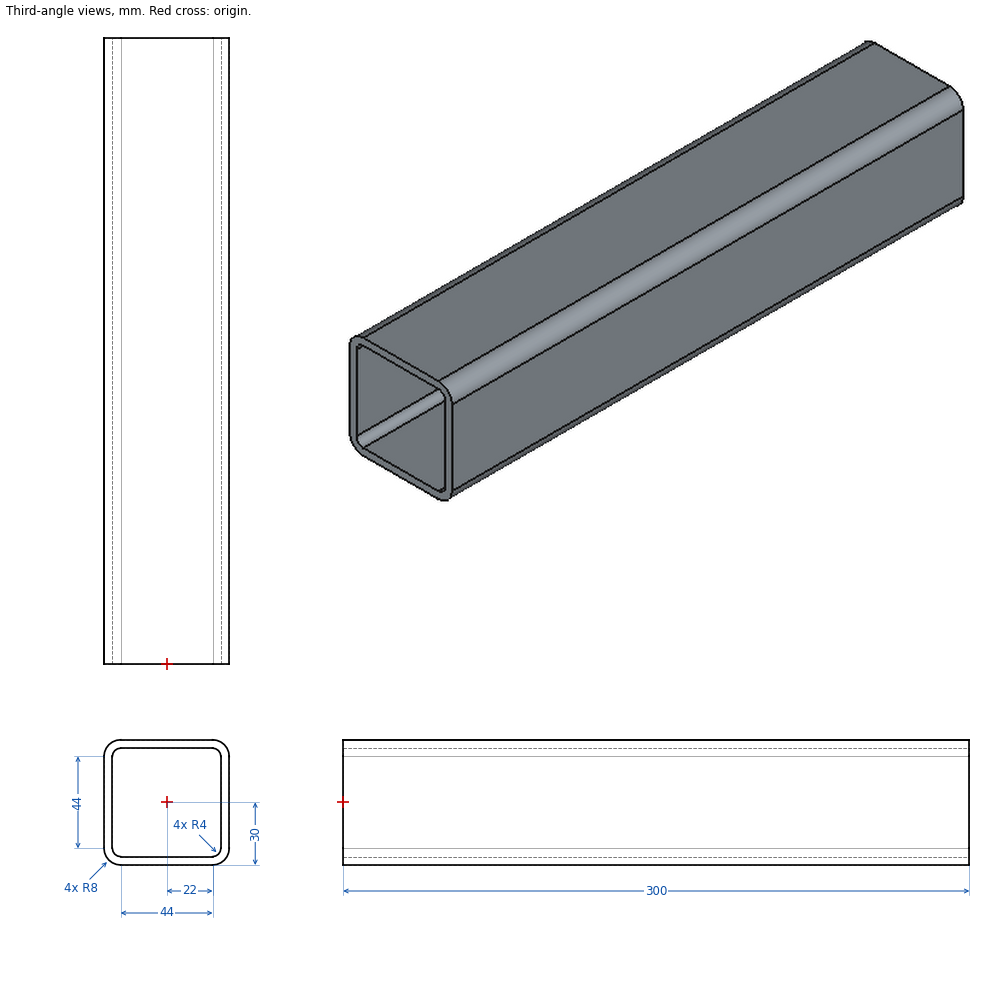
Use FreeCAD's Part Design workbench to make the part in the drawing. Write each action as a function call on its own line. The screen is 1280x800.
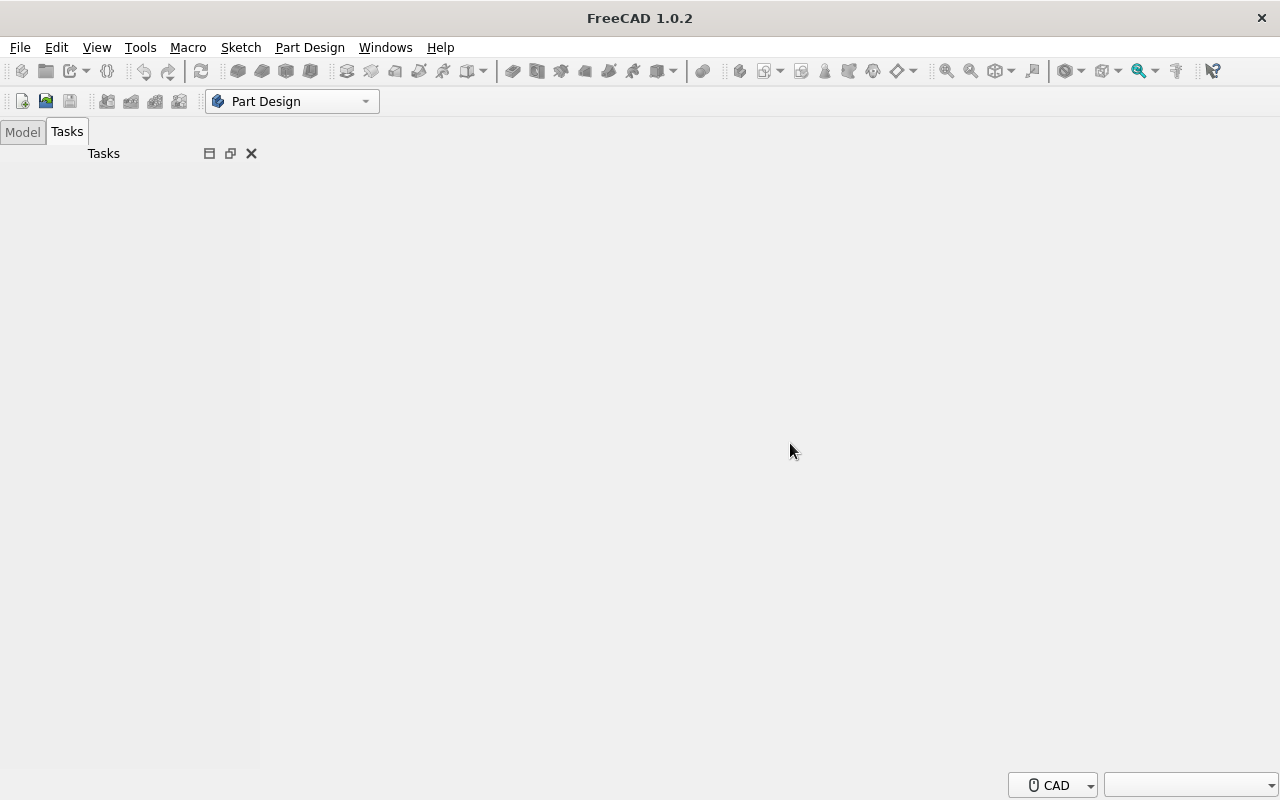
key(ctrl+n)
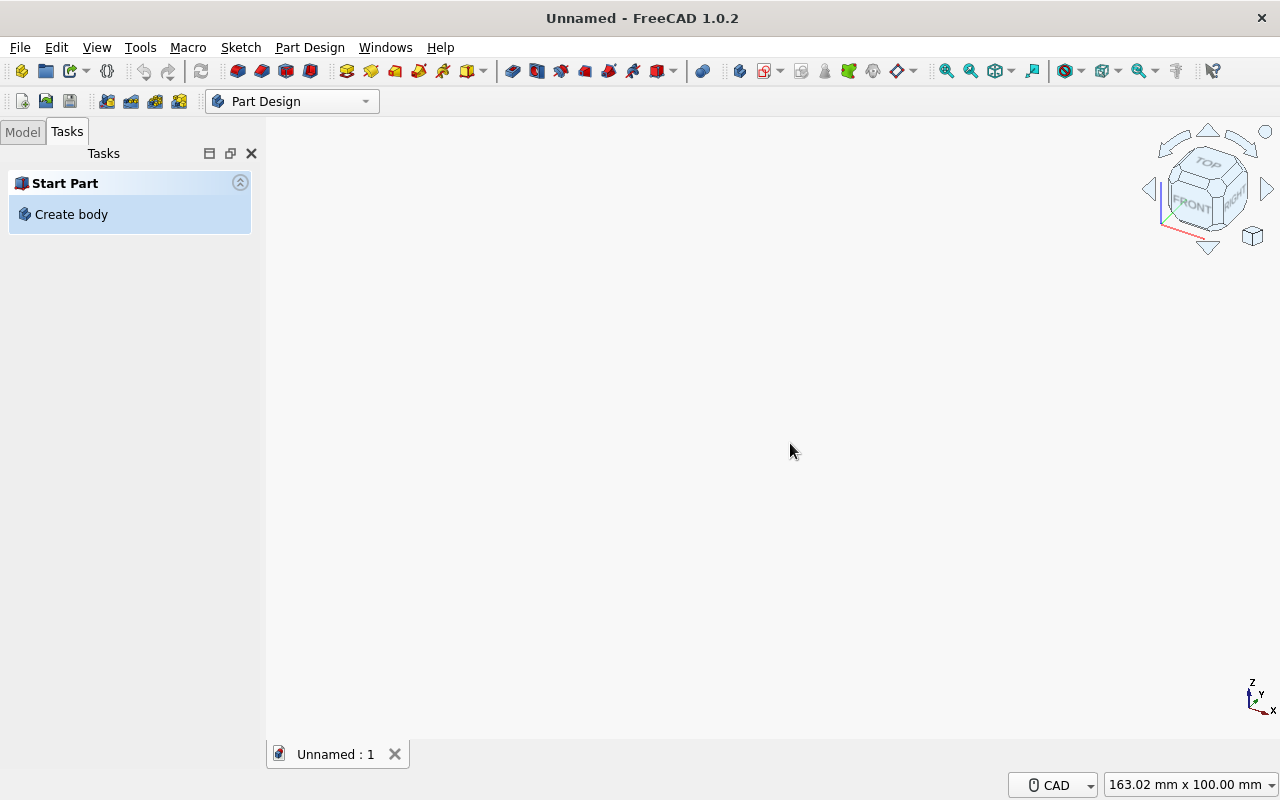
click(764, 72)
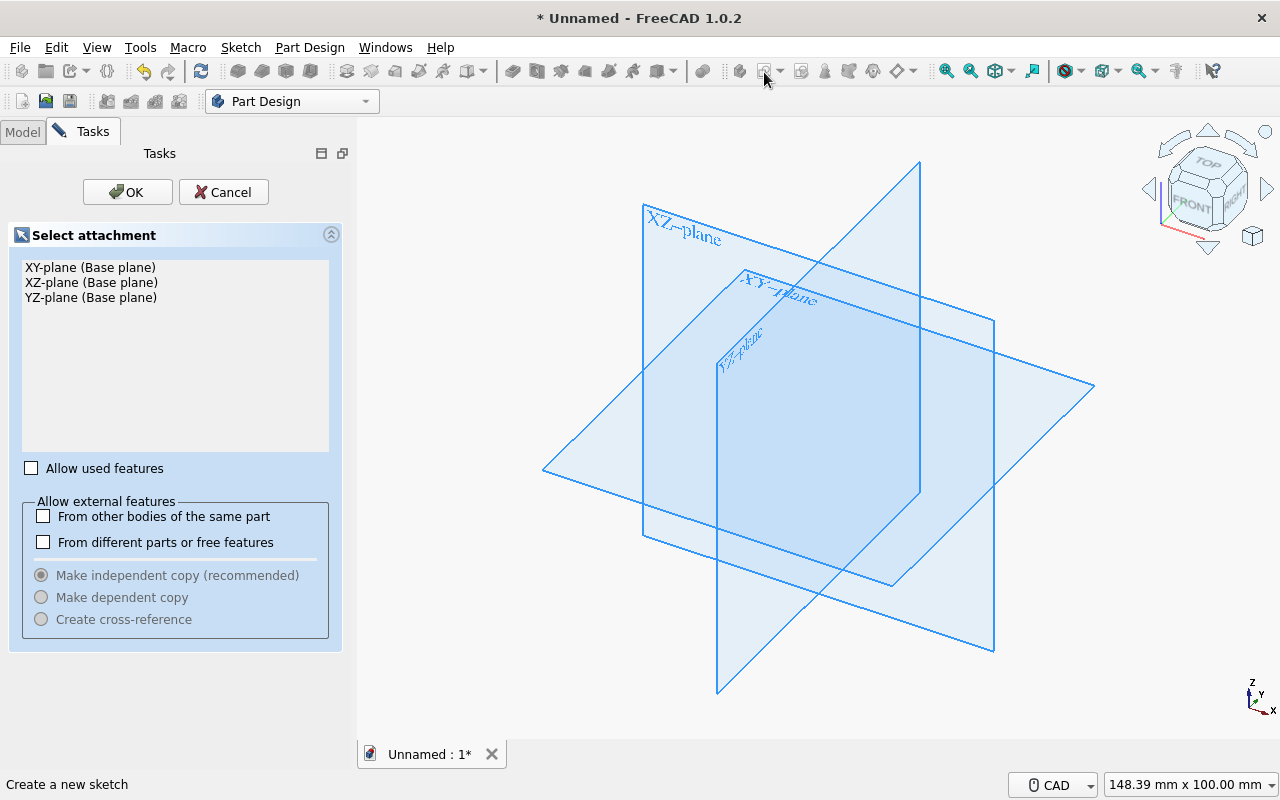
click(82, 282)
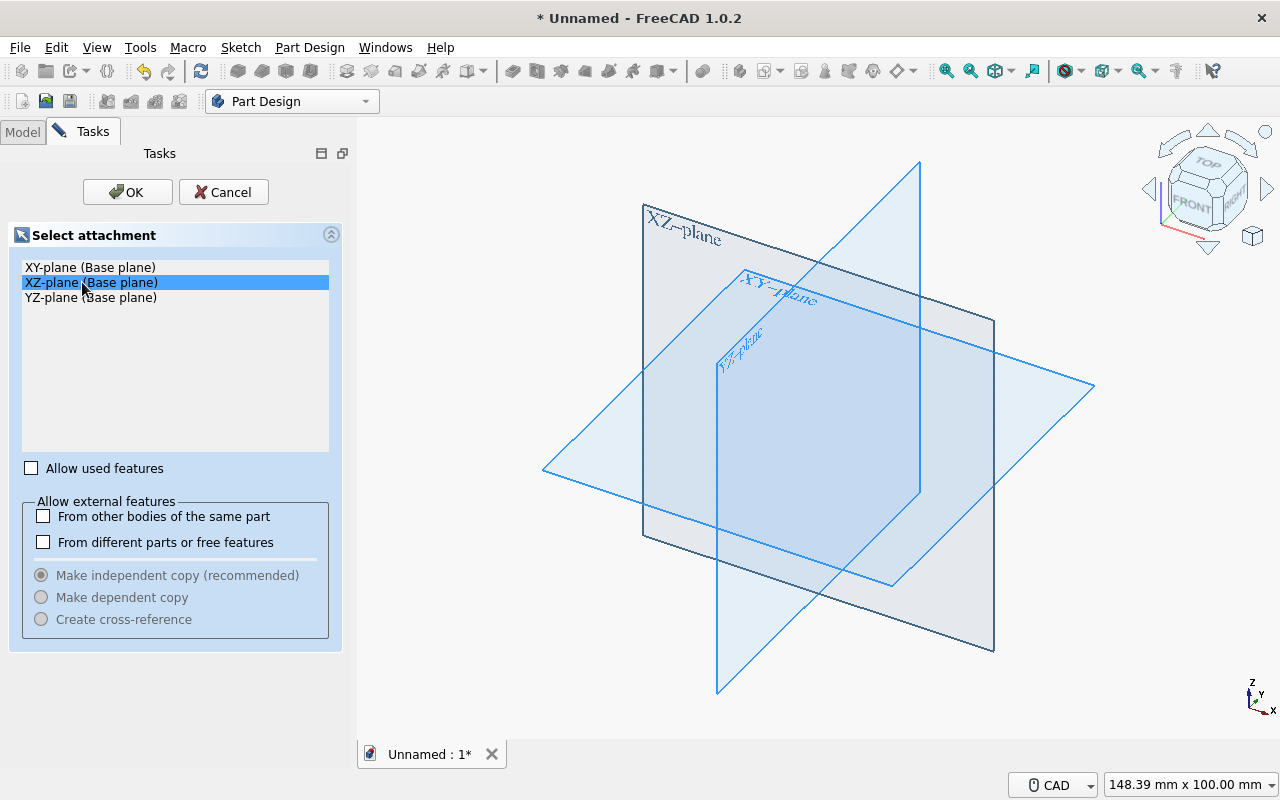
click(128, 192)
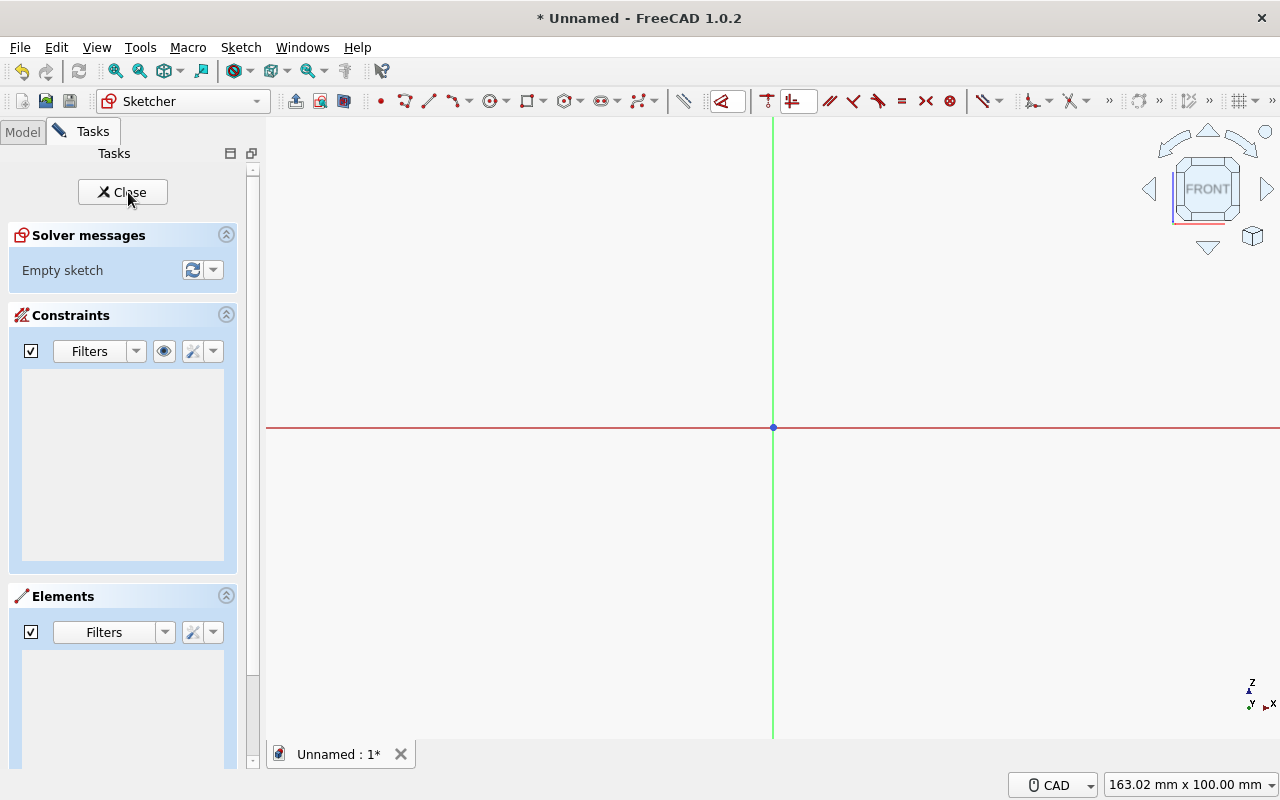
key(g)
key(l)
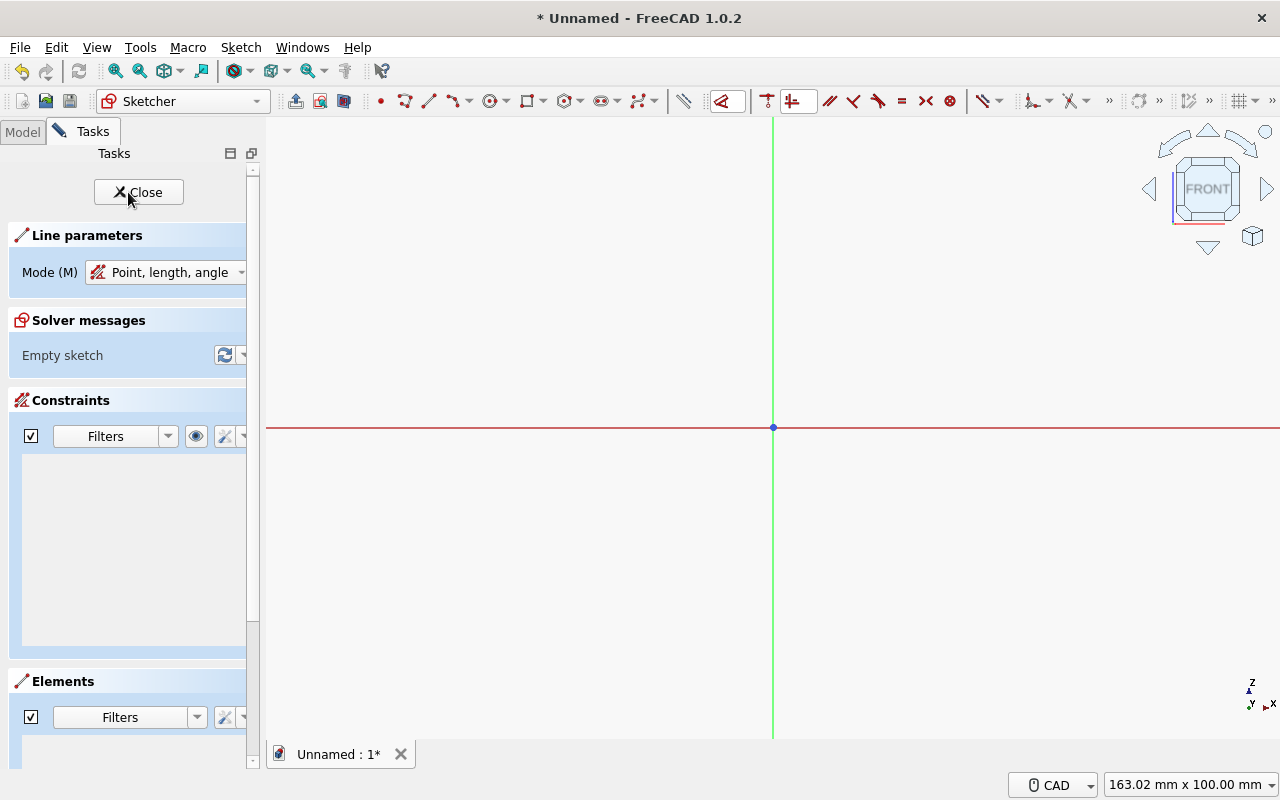
click(910, 615)
click(636, 615)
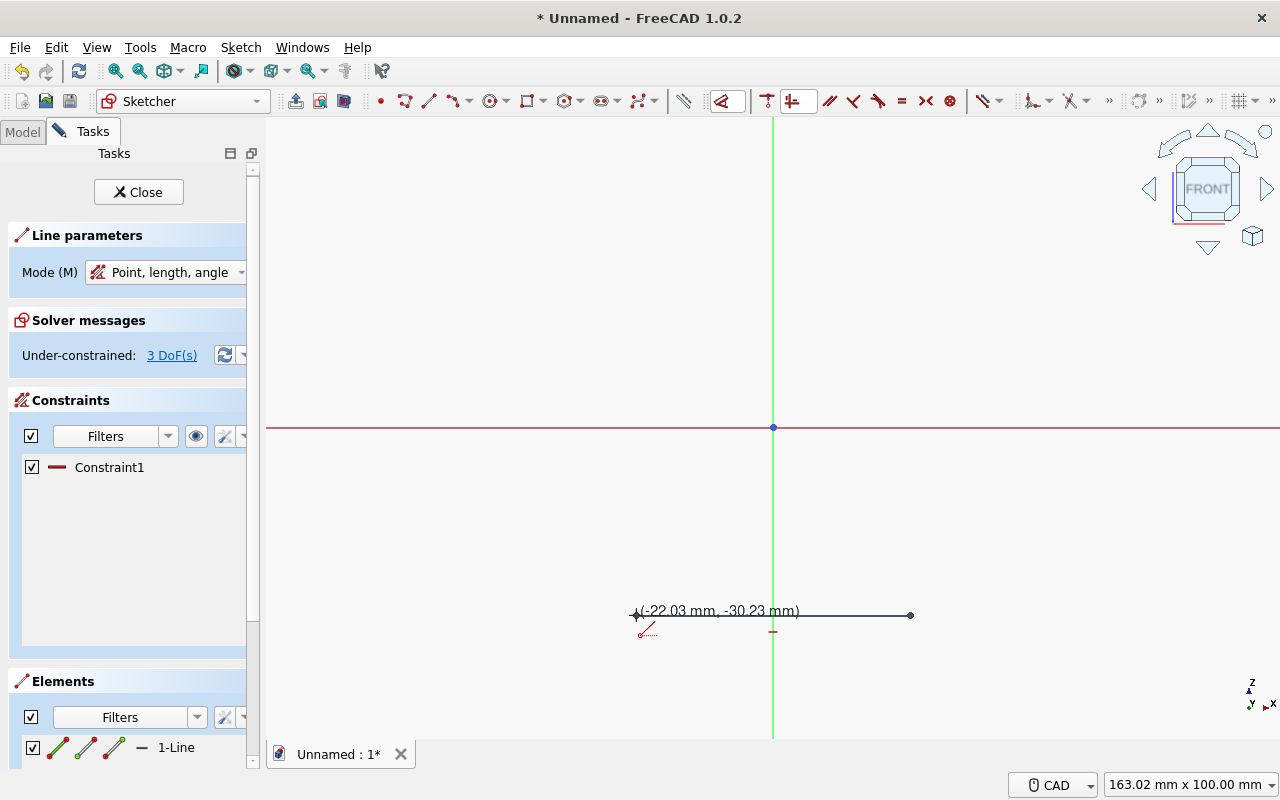
click(586, 565)
click(586, 291)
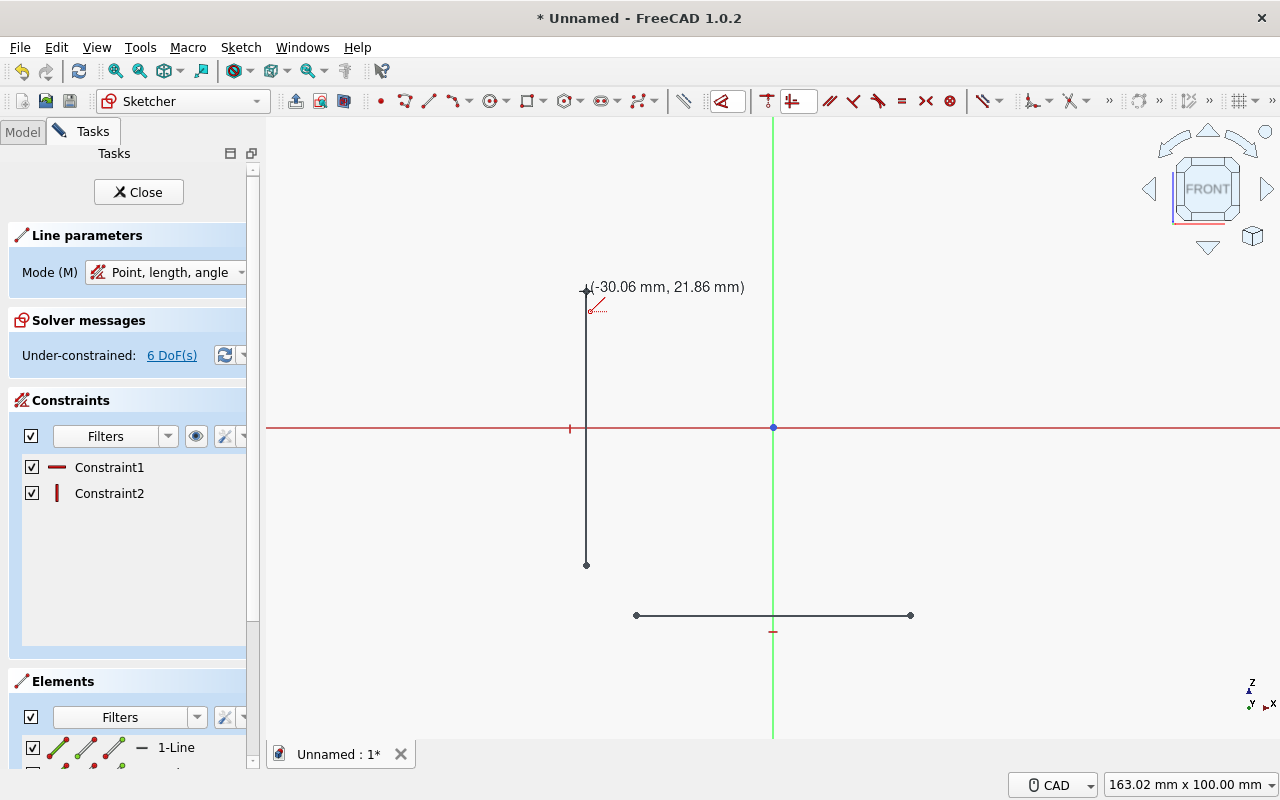
click(636, 241)
click(910, 241)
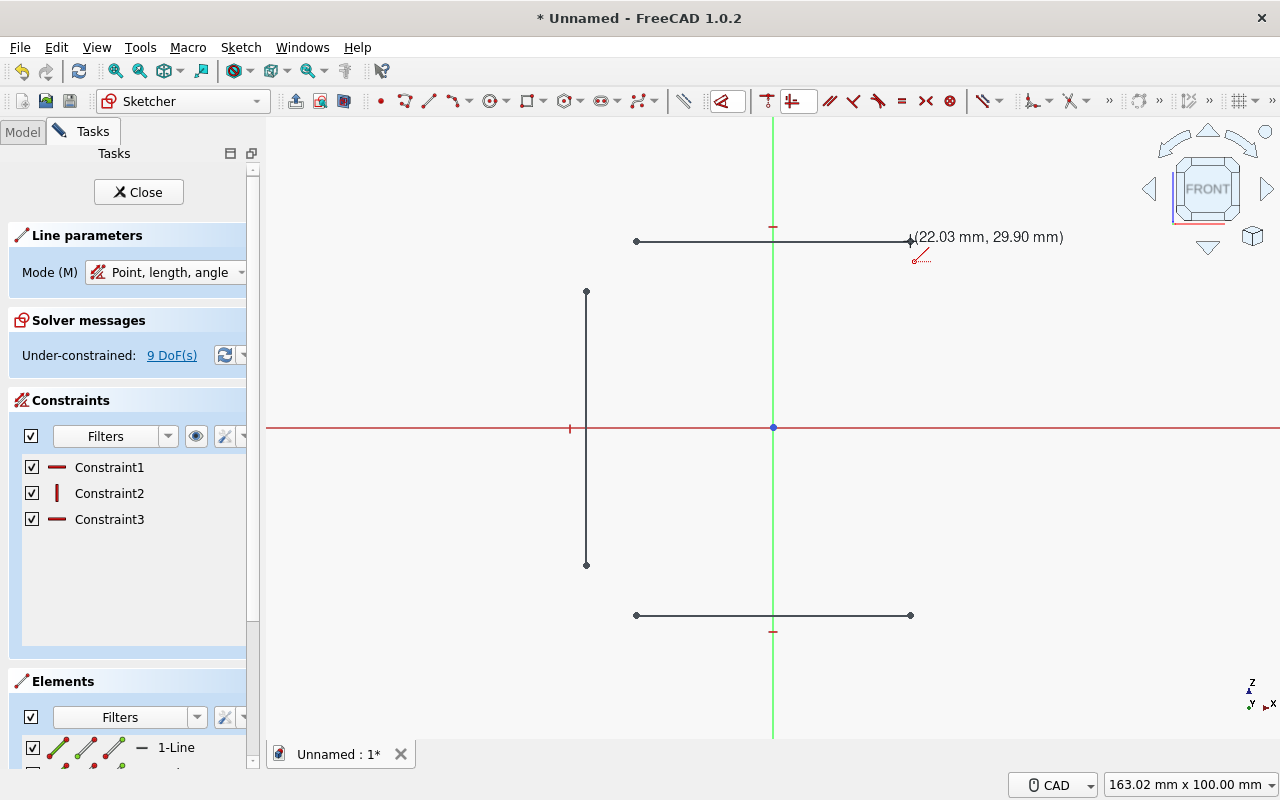
click(960, 291)
click(960, 565)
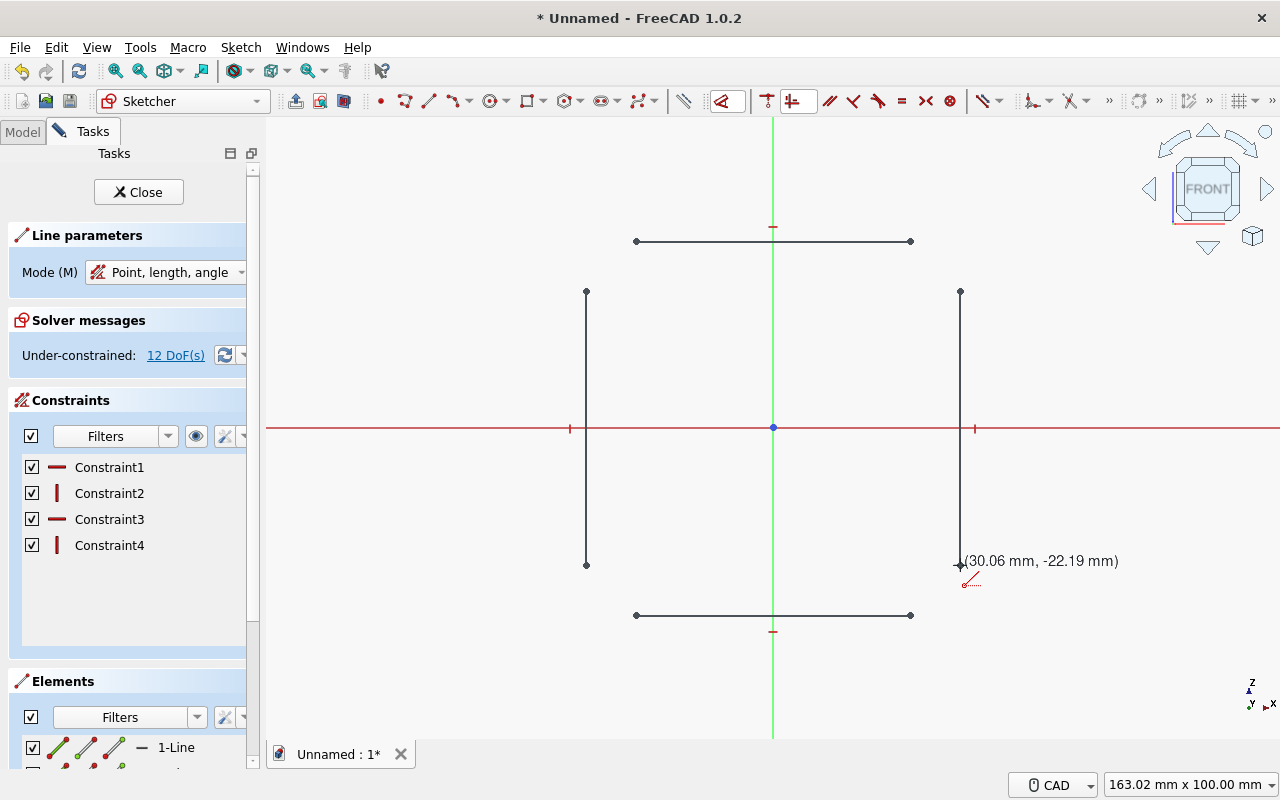
key(g)
key(3)
key(a)